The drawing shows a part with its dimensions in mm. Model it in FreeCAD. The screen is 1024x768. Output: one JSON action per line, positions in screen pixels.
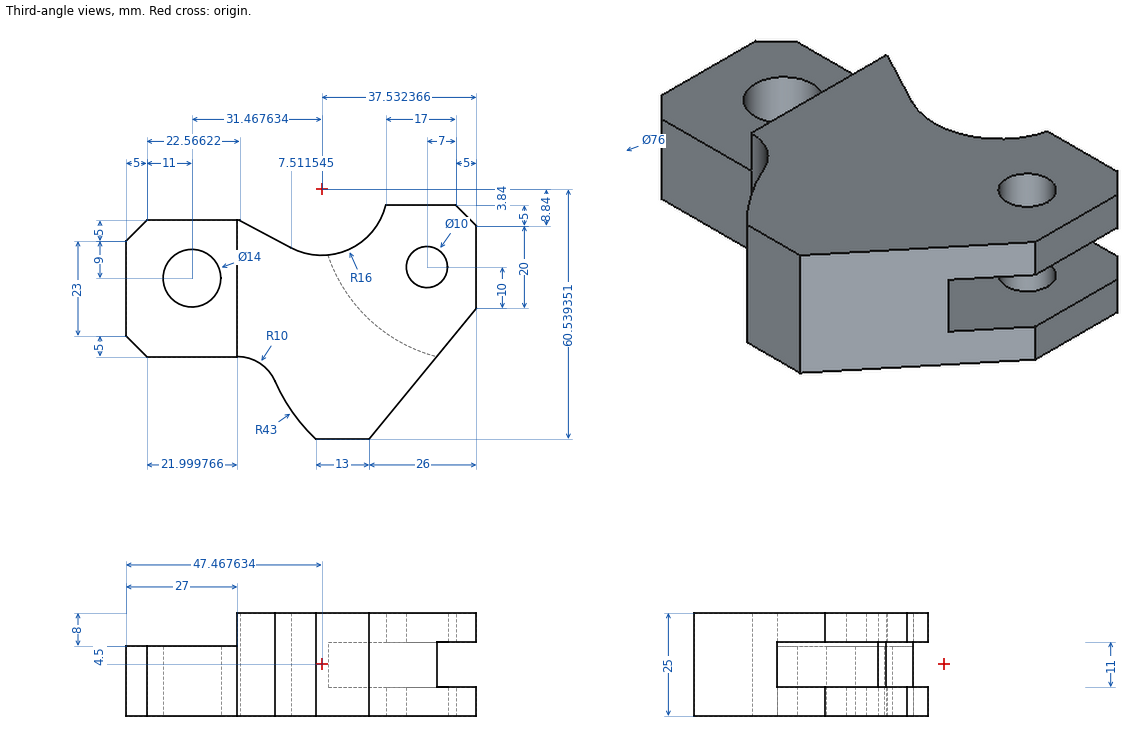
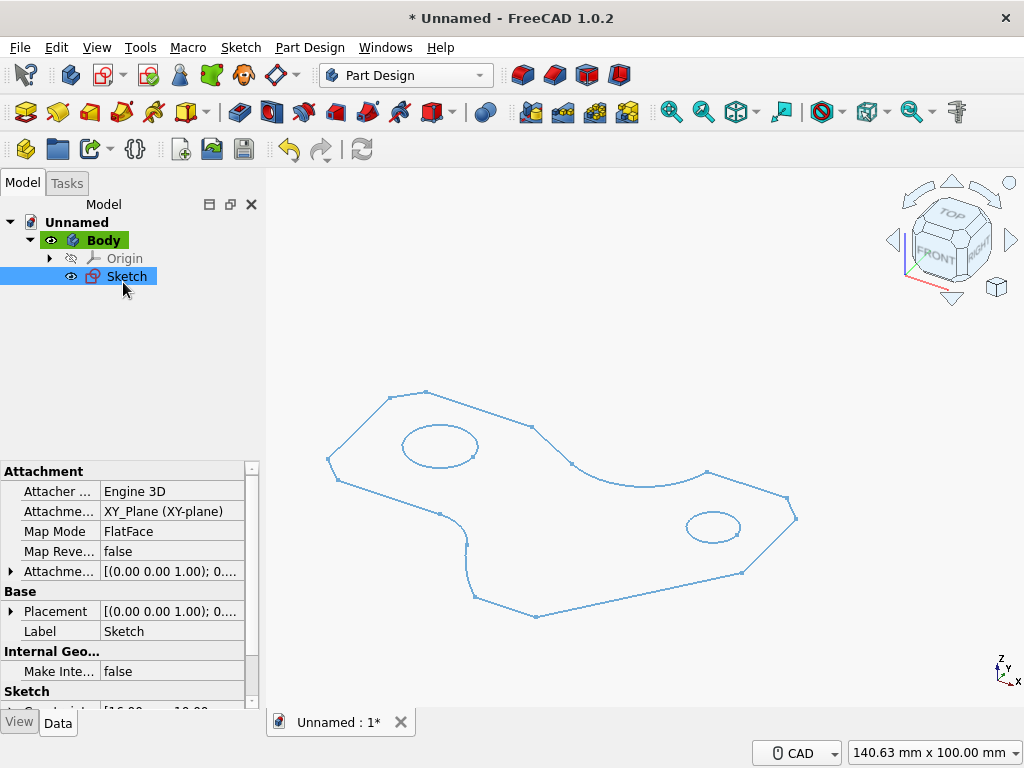
{"action": "left_click", "coordinate": [26, 112]}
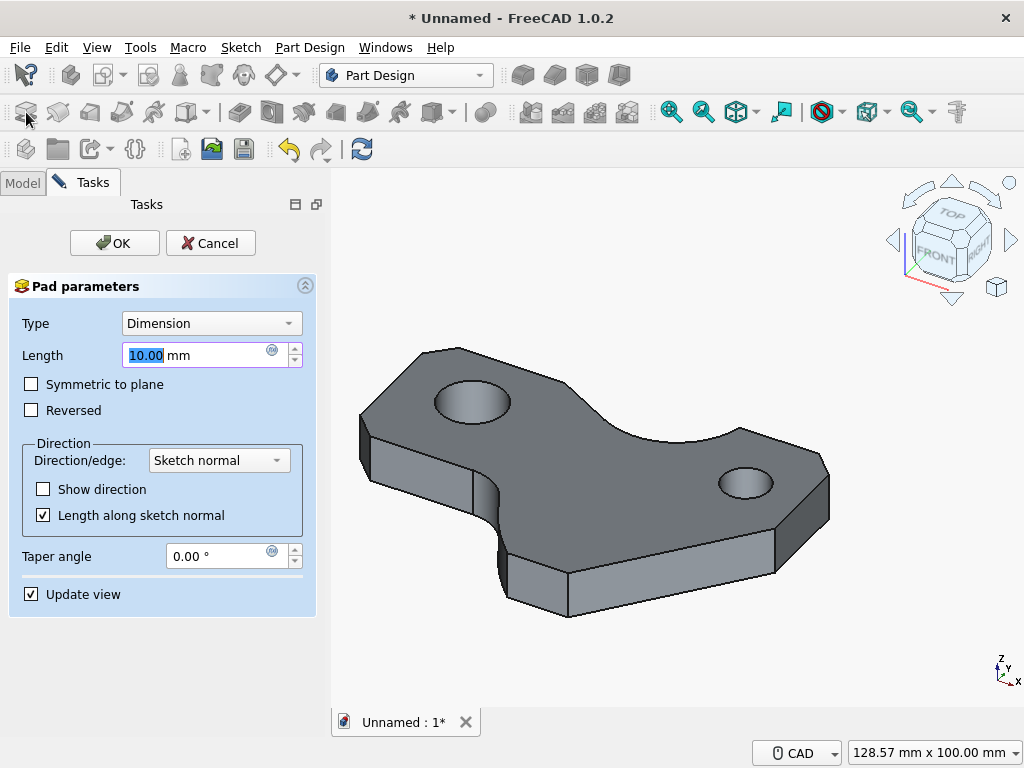
{"action": "type", "text": "25"}
{"action": "key", "text": "Tab"}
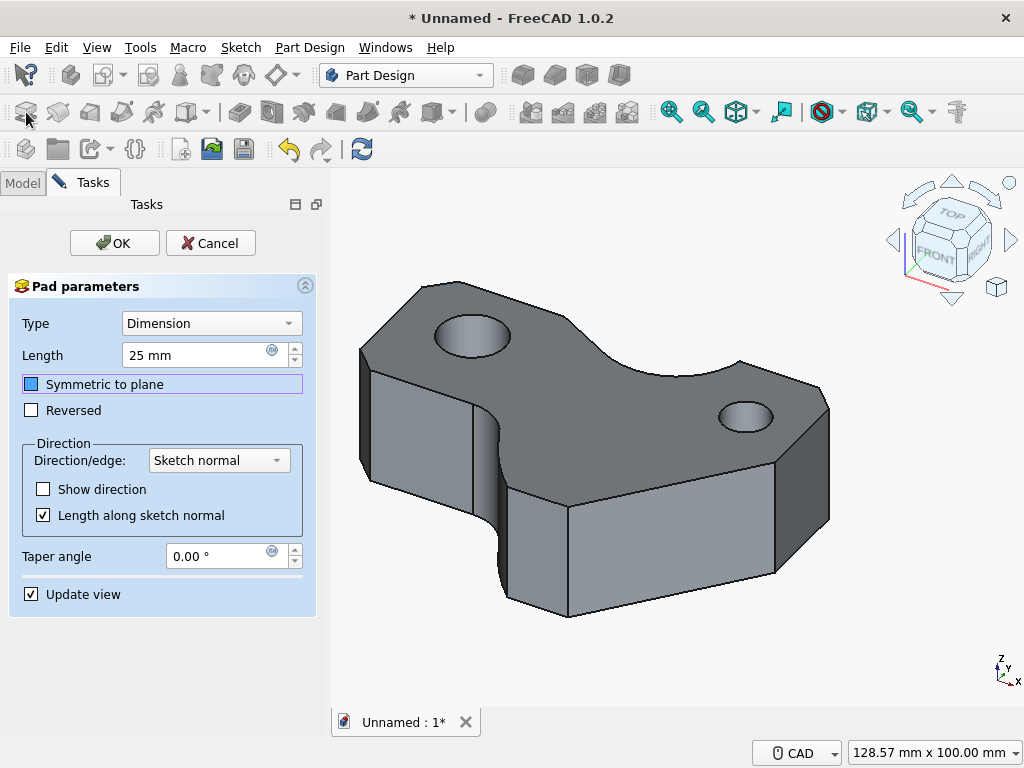
{"action": "left_click", "coordinate": [30, 384]}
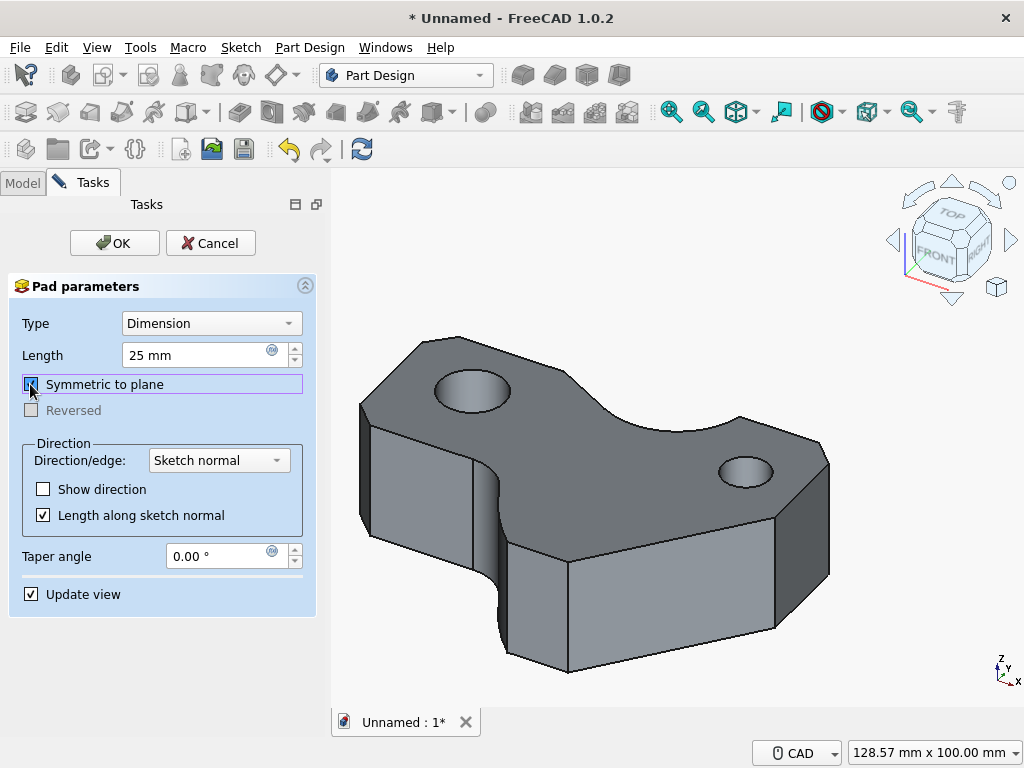
{"action": "left_click", "coordinate": [115, 243]}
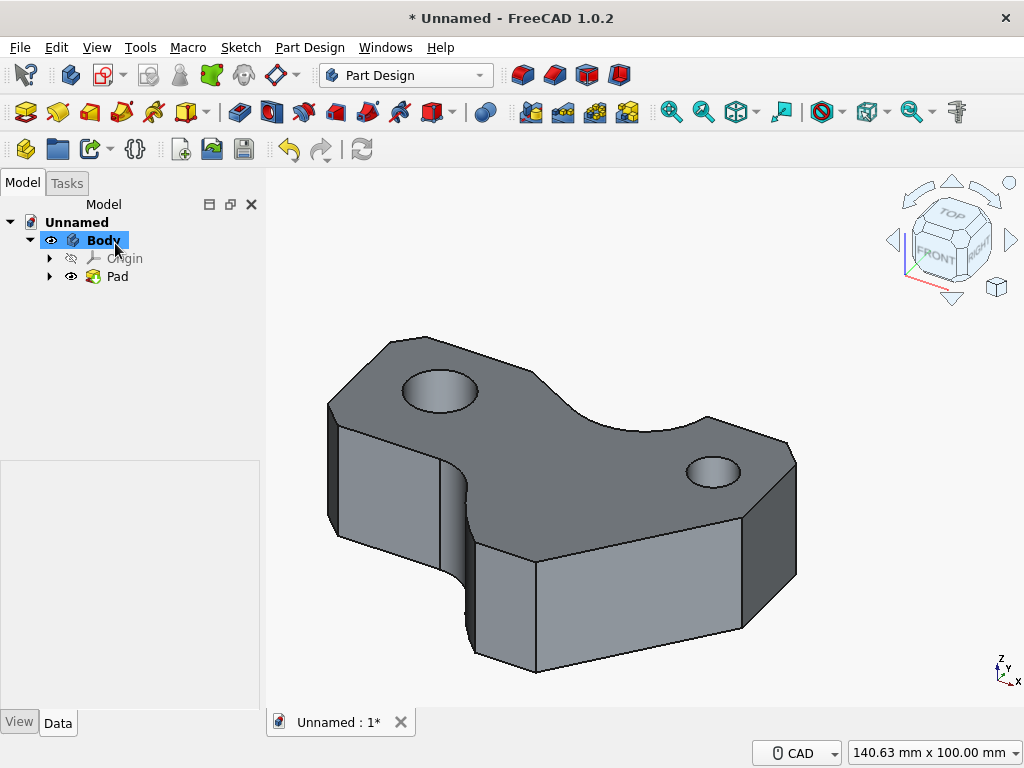
{"action": "left_click", "coordinate": [672, 112]}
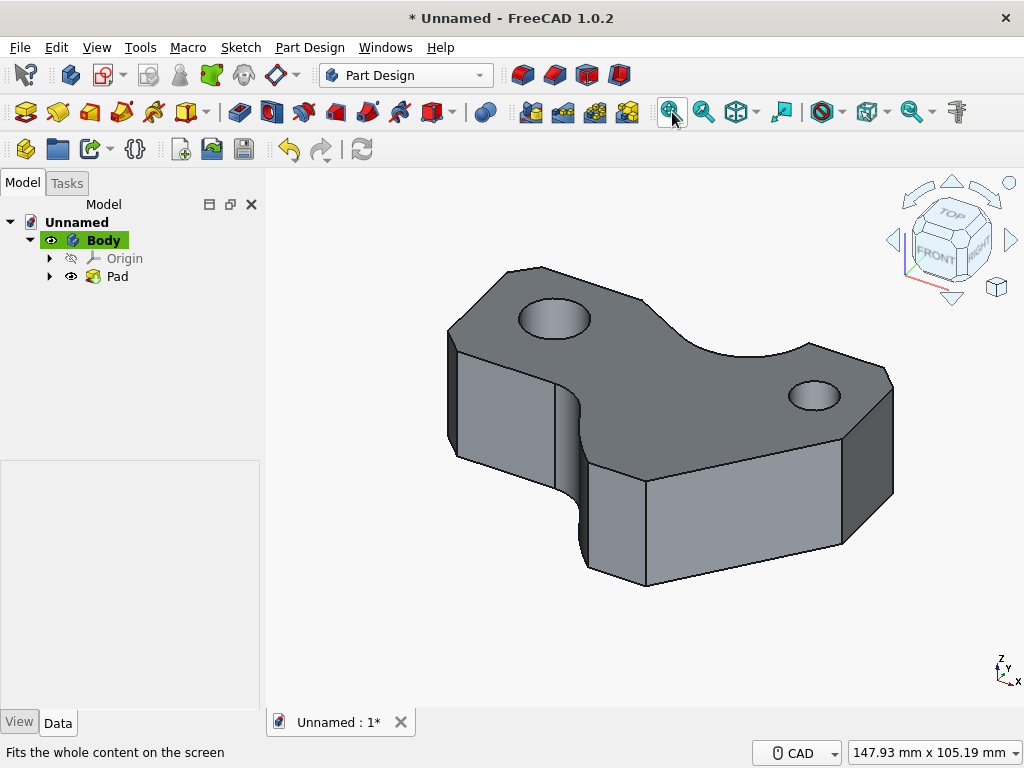
{"action": "left_click", "coordinate": [104, 76]}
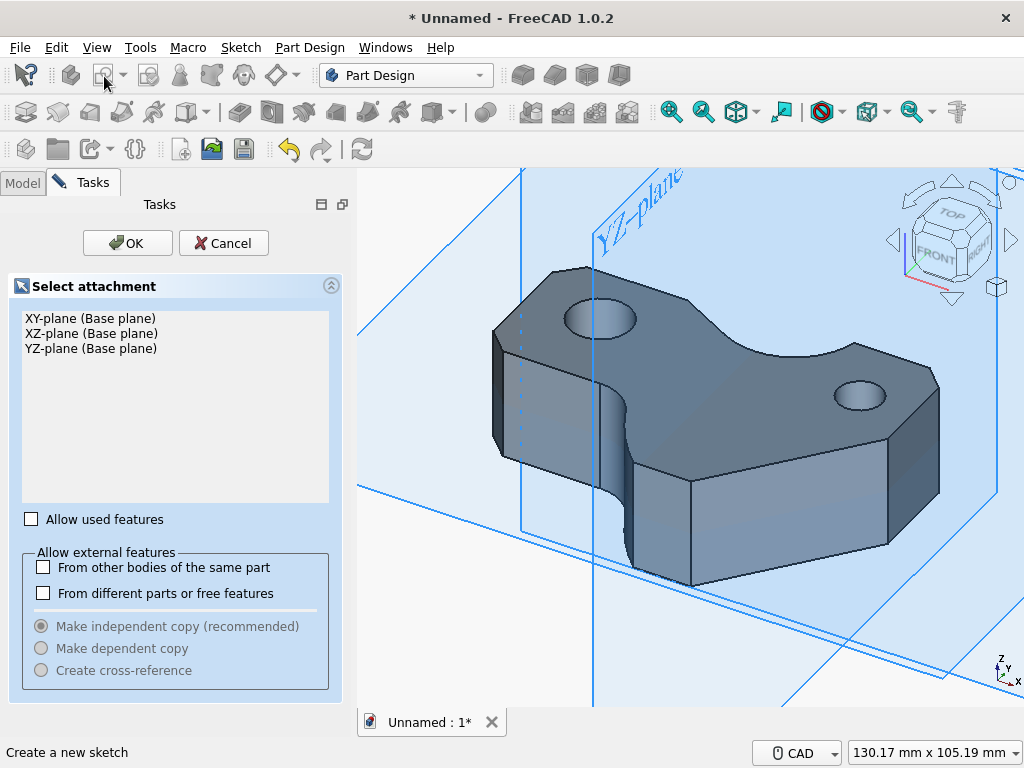
{"action": "left_click", "coordinate": [82, 334]}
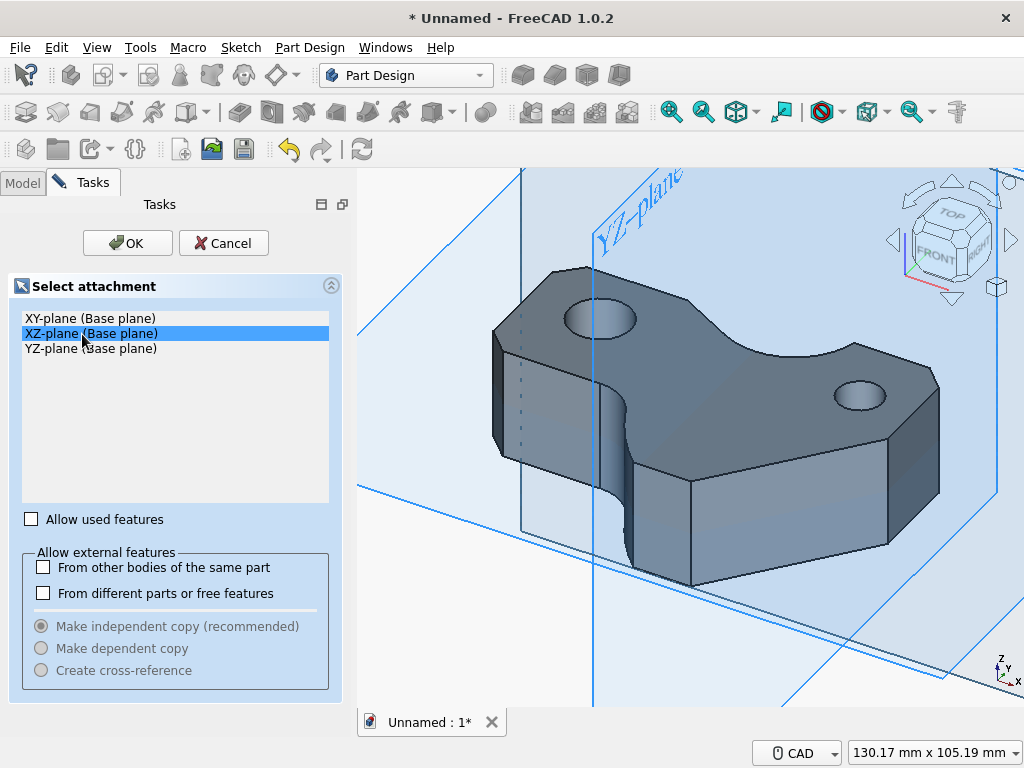
{"action": "left_click", "coordinate": [128, 243]}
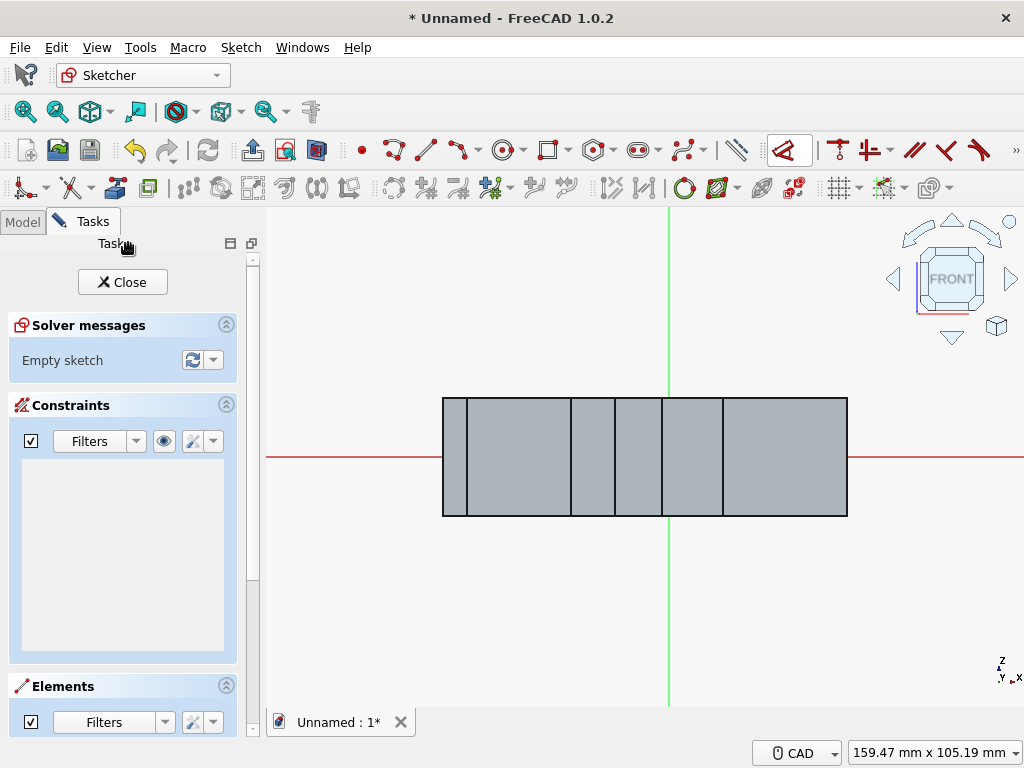
{"action": "left_click", "coordinate": [318, 150]}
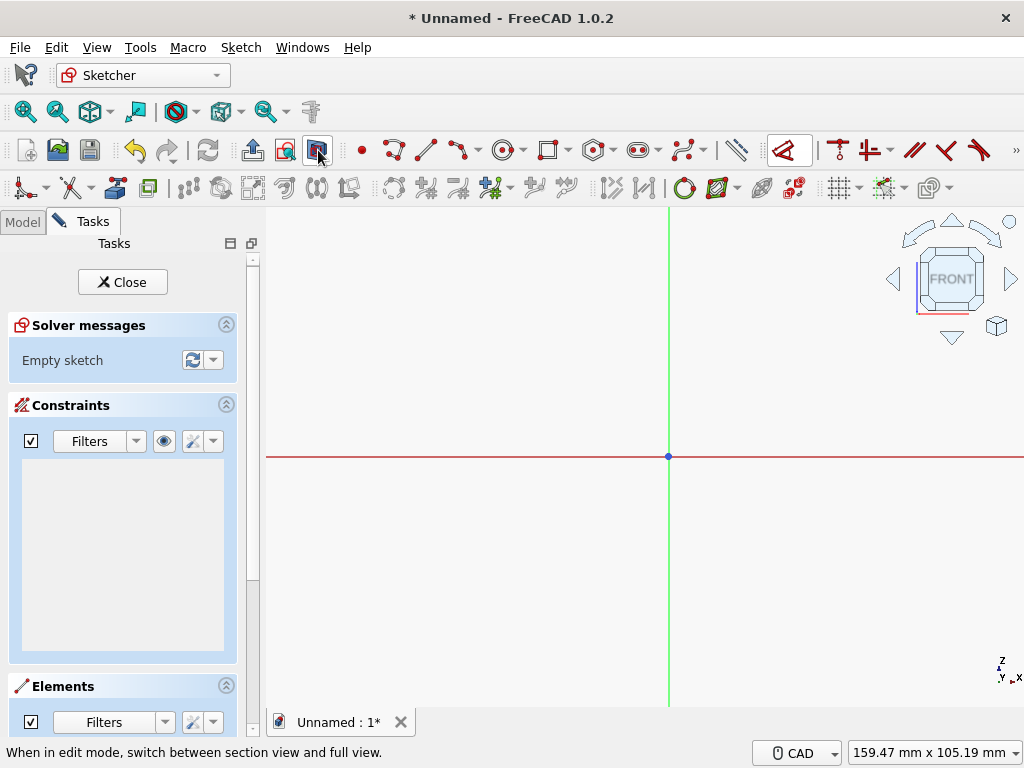
{"action": "scroll", "coordinate": [531, 391], "scroll_direction": "up", "scroll_amount": 3}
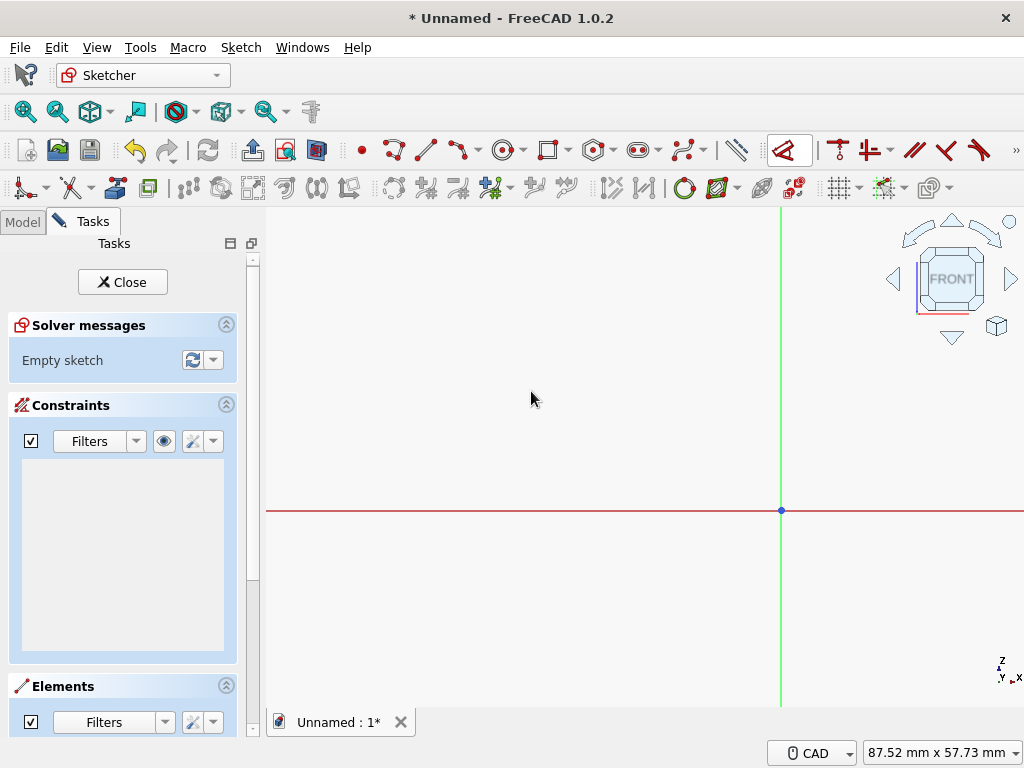
{"action": "left_click", "coordinate": [548, 150]}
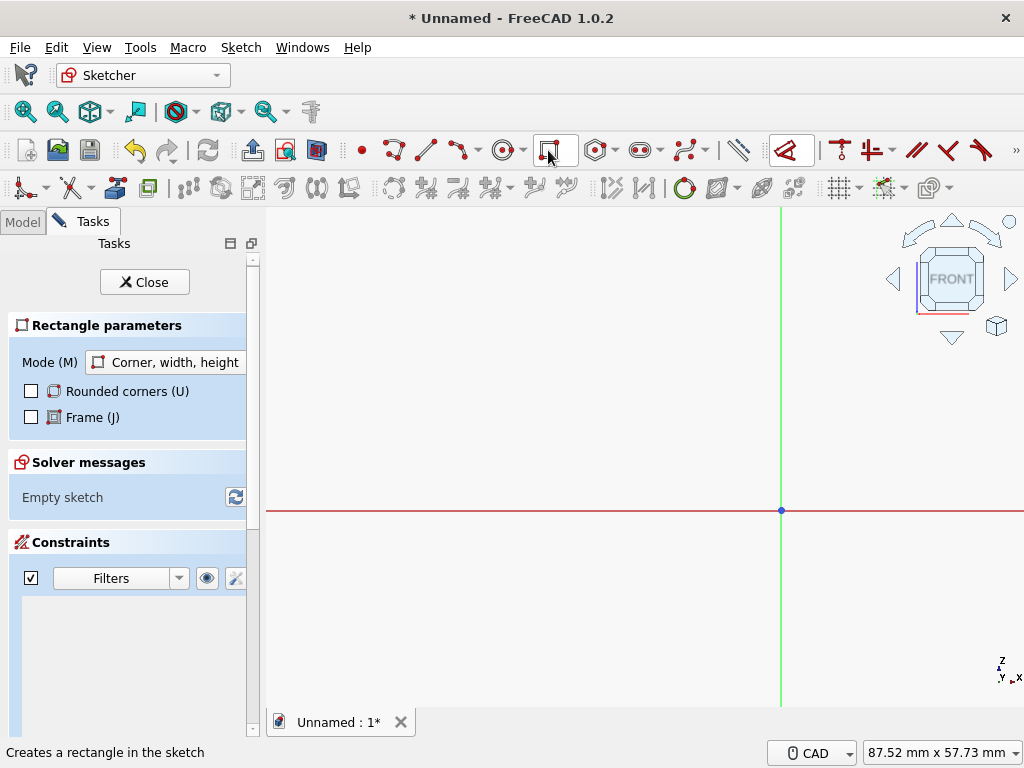
{"action": "left_click", "coordinate": [370, 403]}
{"action": "left_click", "coordinate": [604, 472]}
{"action": "key", "text": "Escape"}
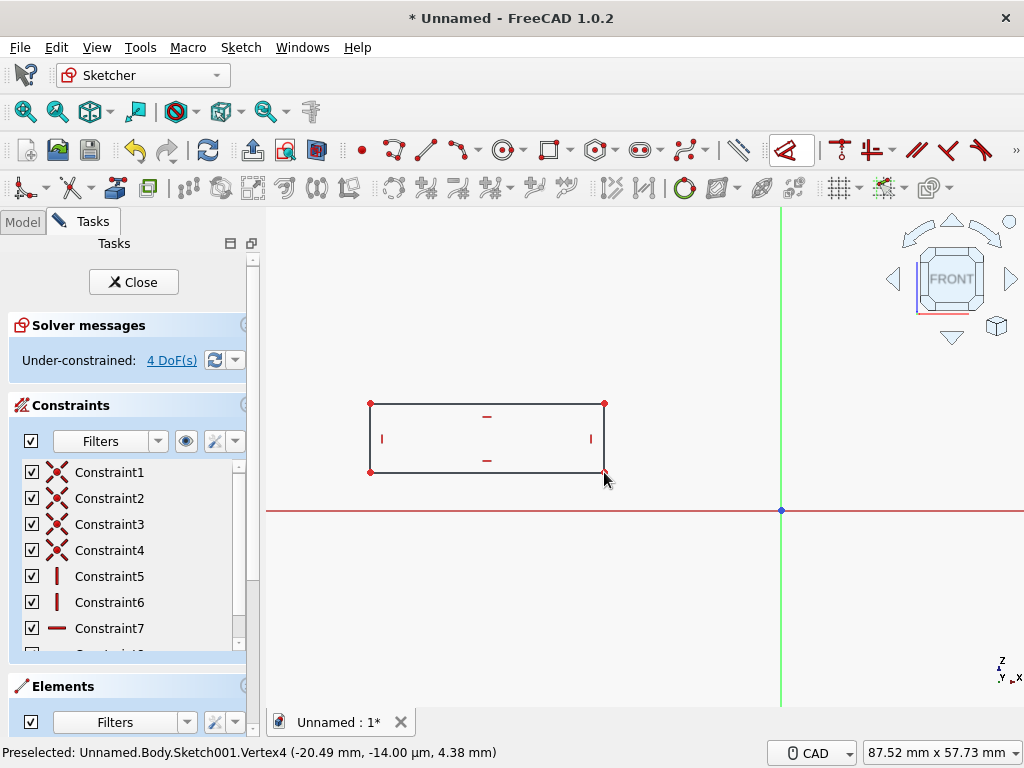
{"action": "left_click", "coordinate": [370, 425]}